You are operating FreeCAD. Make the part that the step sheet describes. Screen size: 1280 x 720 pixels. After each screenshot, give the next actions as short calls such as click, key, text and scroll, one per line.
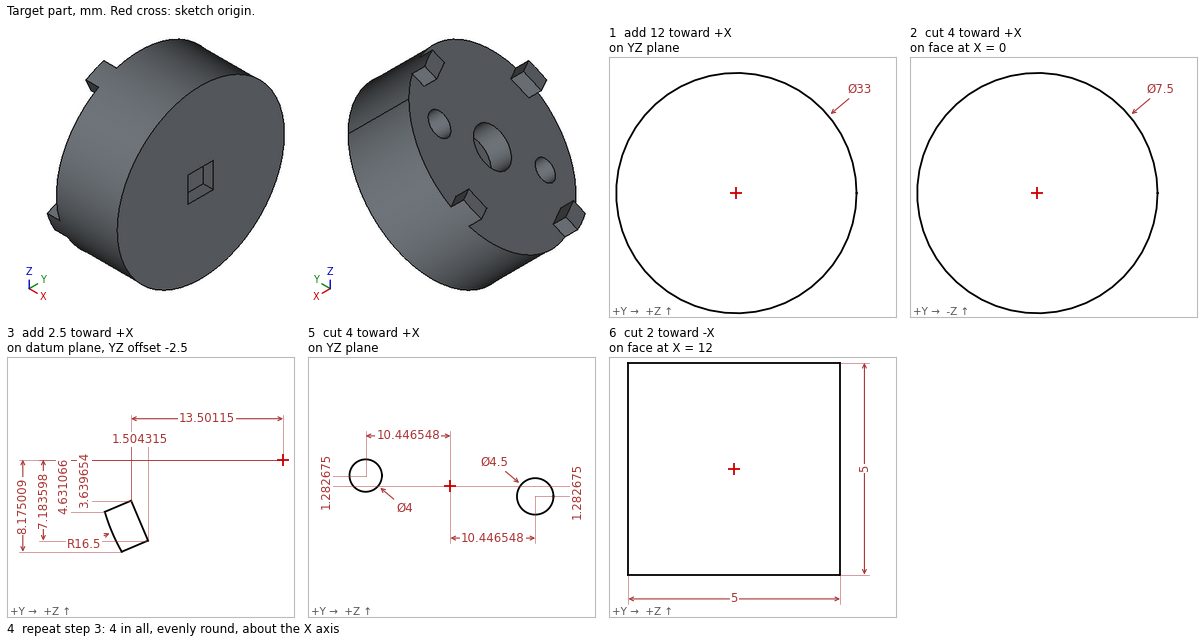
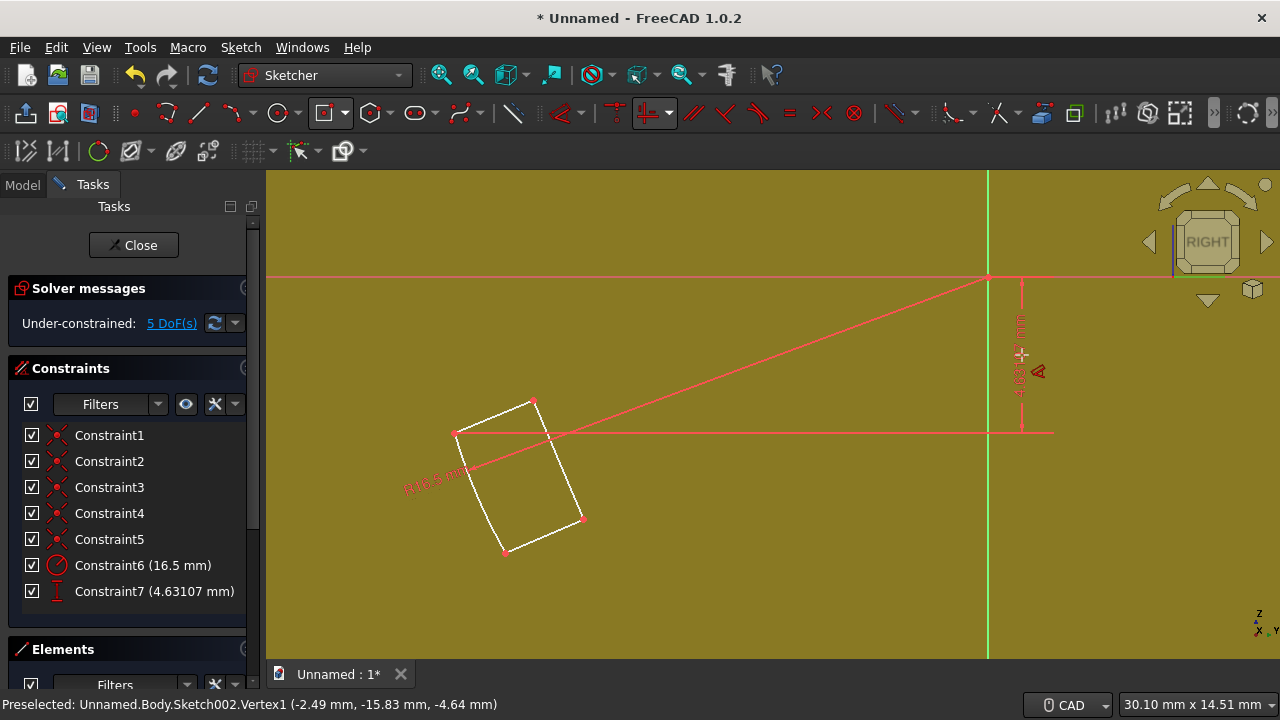
click(533, 400)
click(761, 243)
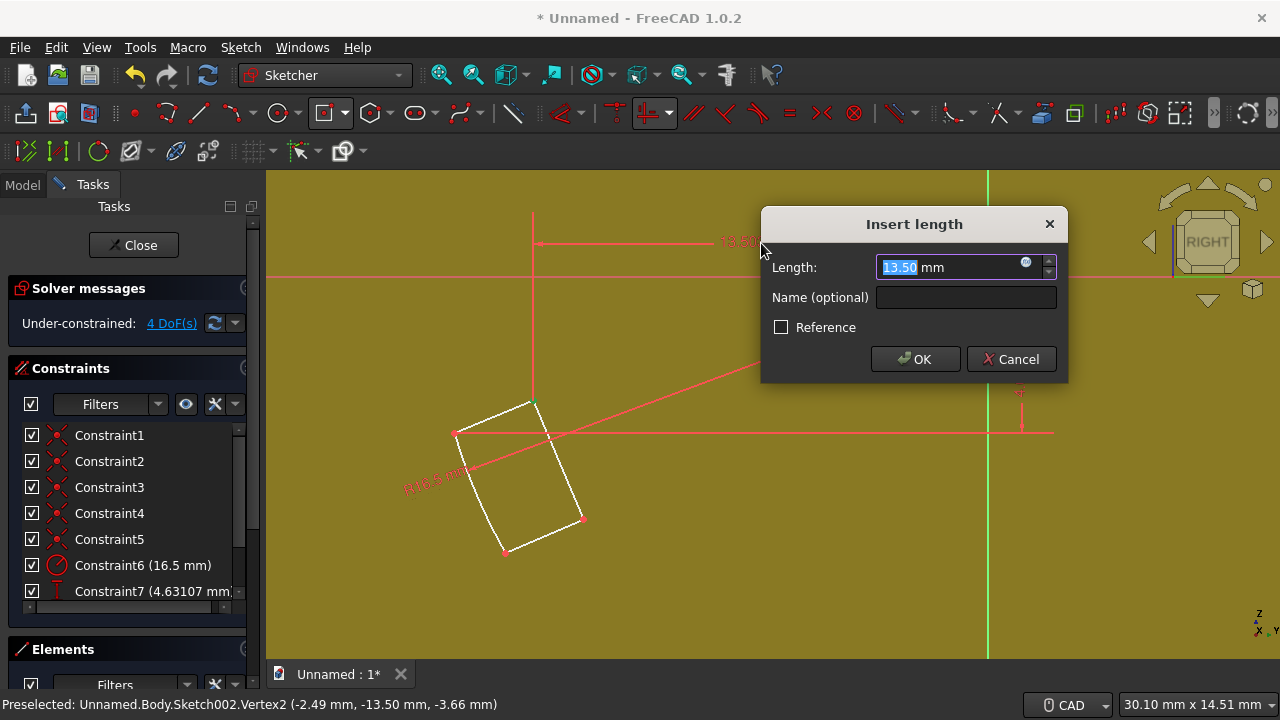
text(13.50115)
key(Return)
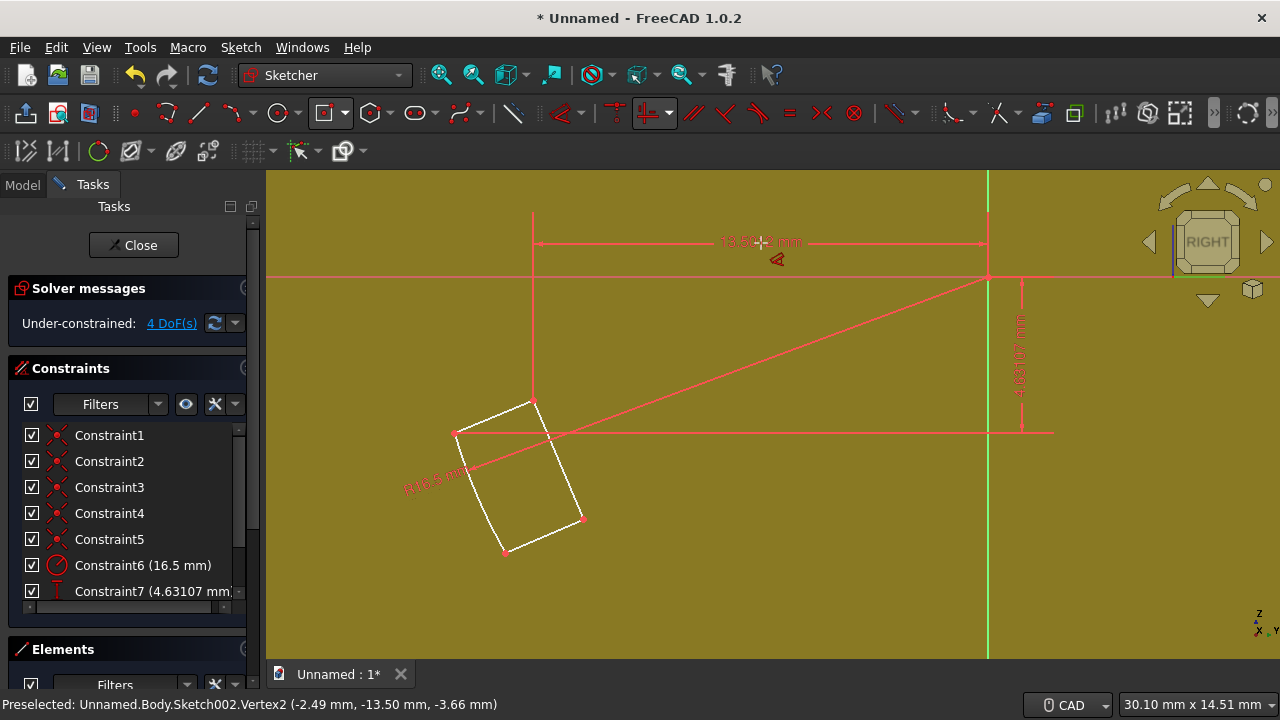
click(533, 400)
click(1022, 310)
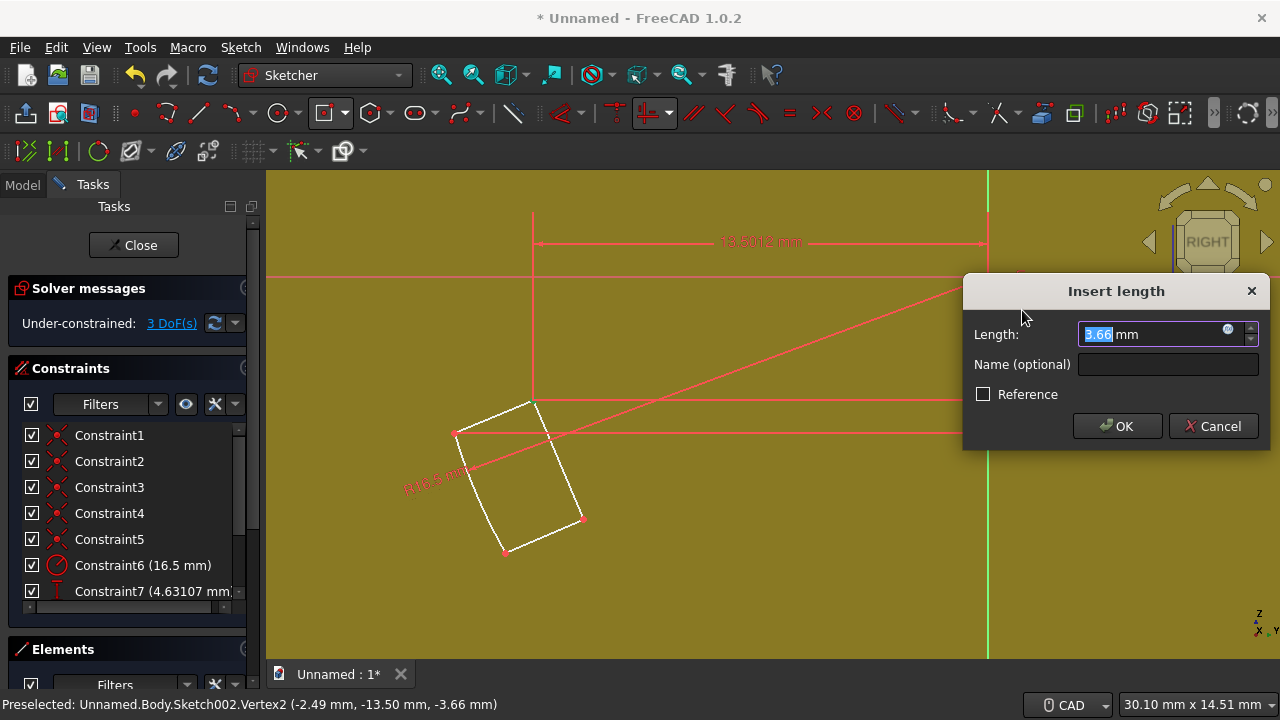
text(3.639654)
key(Return)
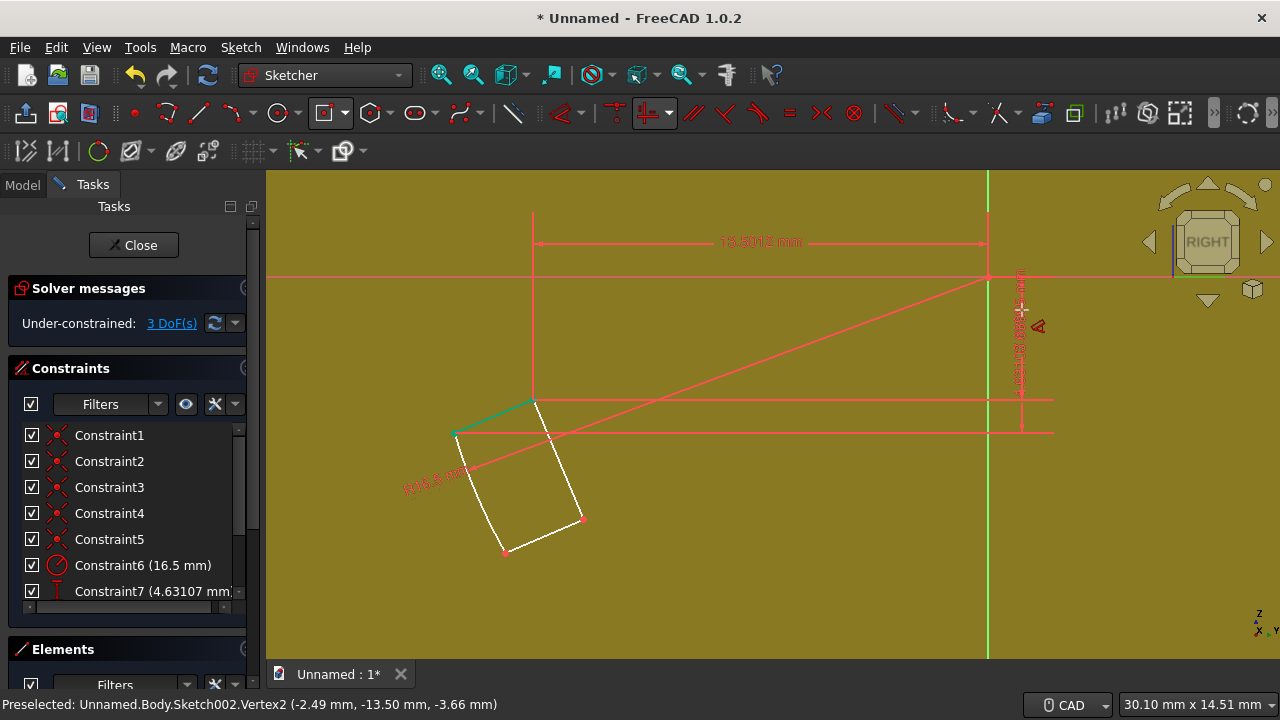
click(584, 520)
click(1022, 398)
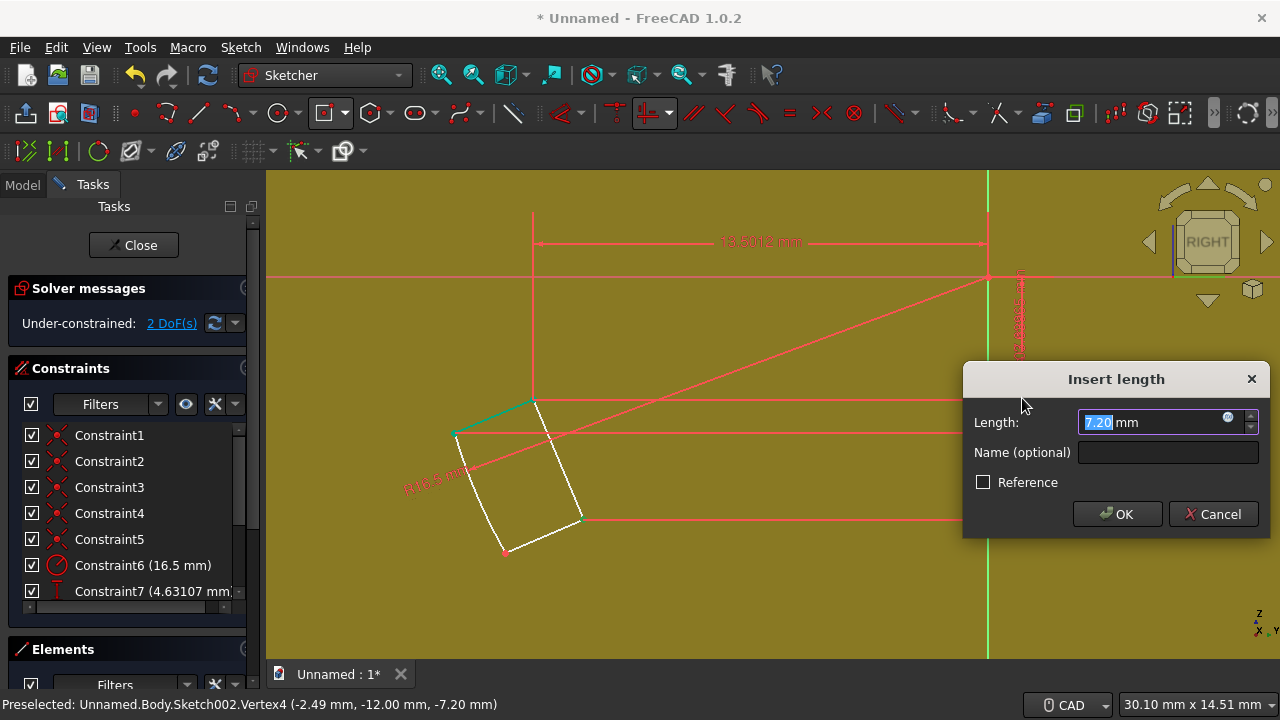
text(7.183598)
key(Return)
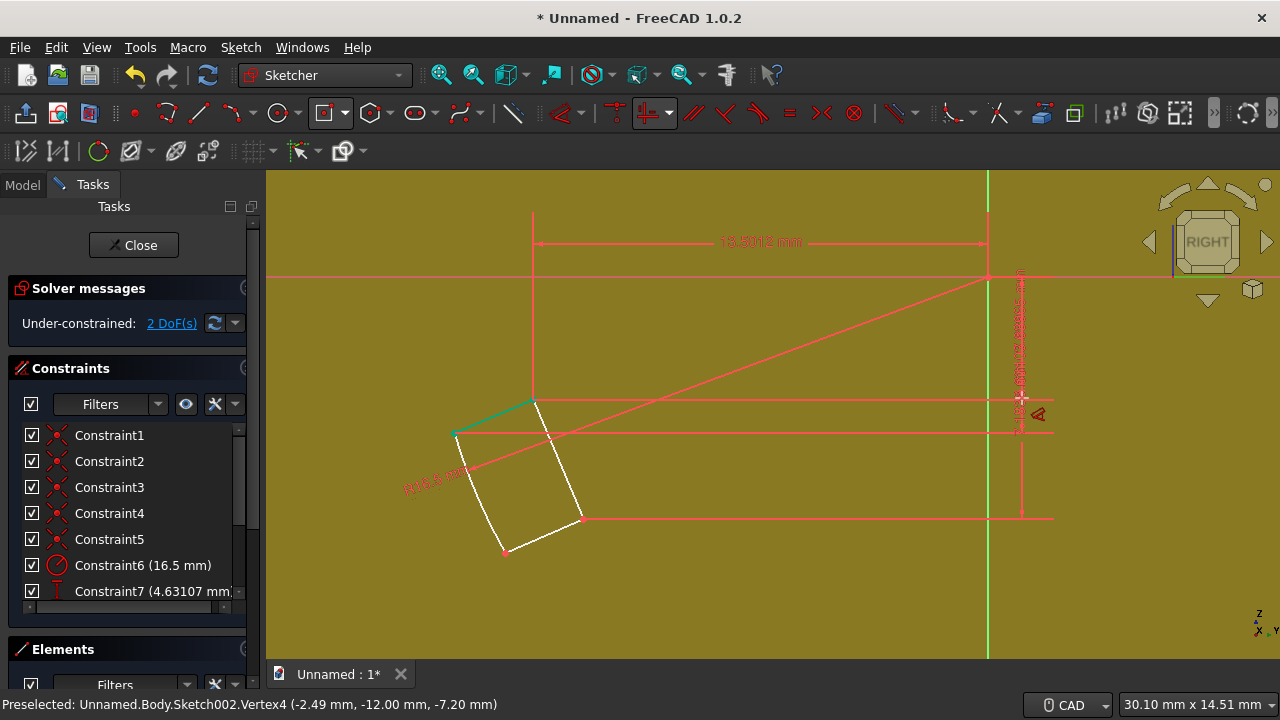
click(506, 553)
click(1022, 479)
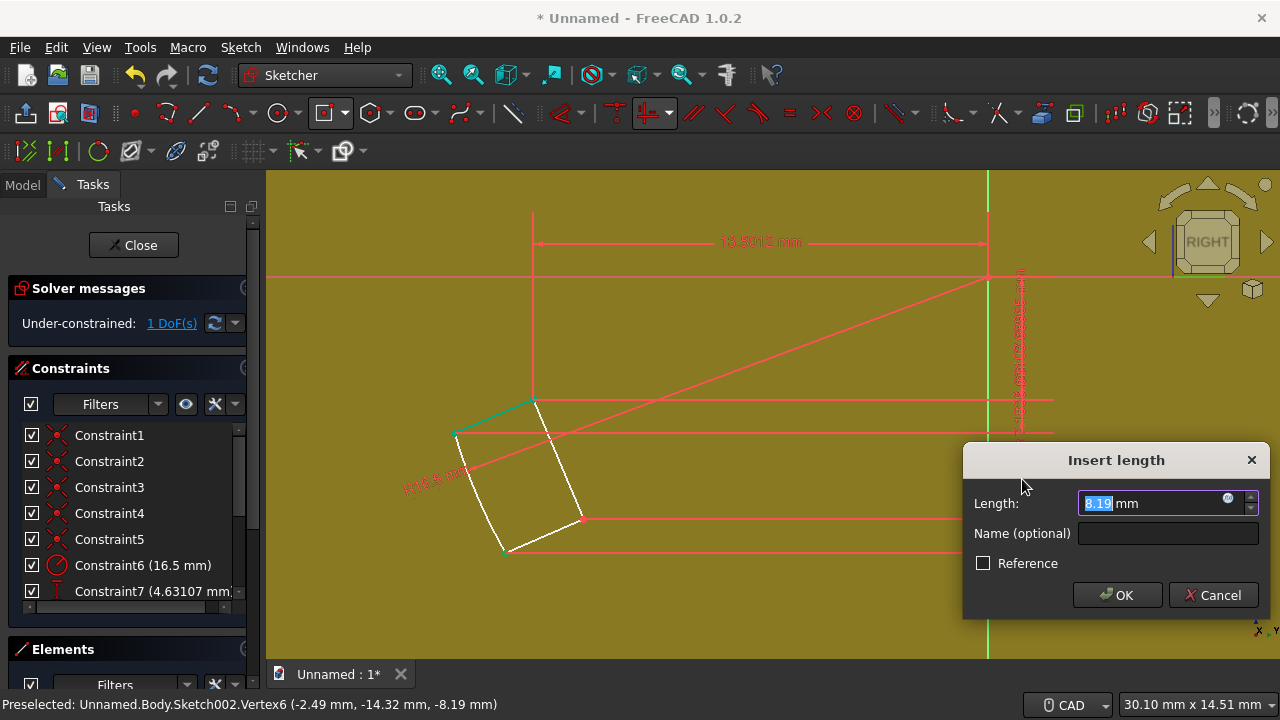
text(8.175009)
key(Return)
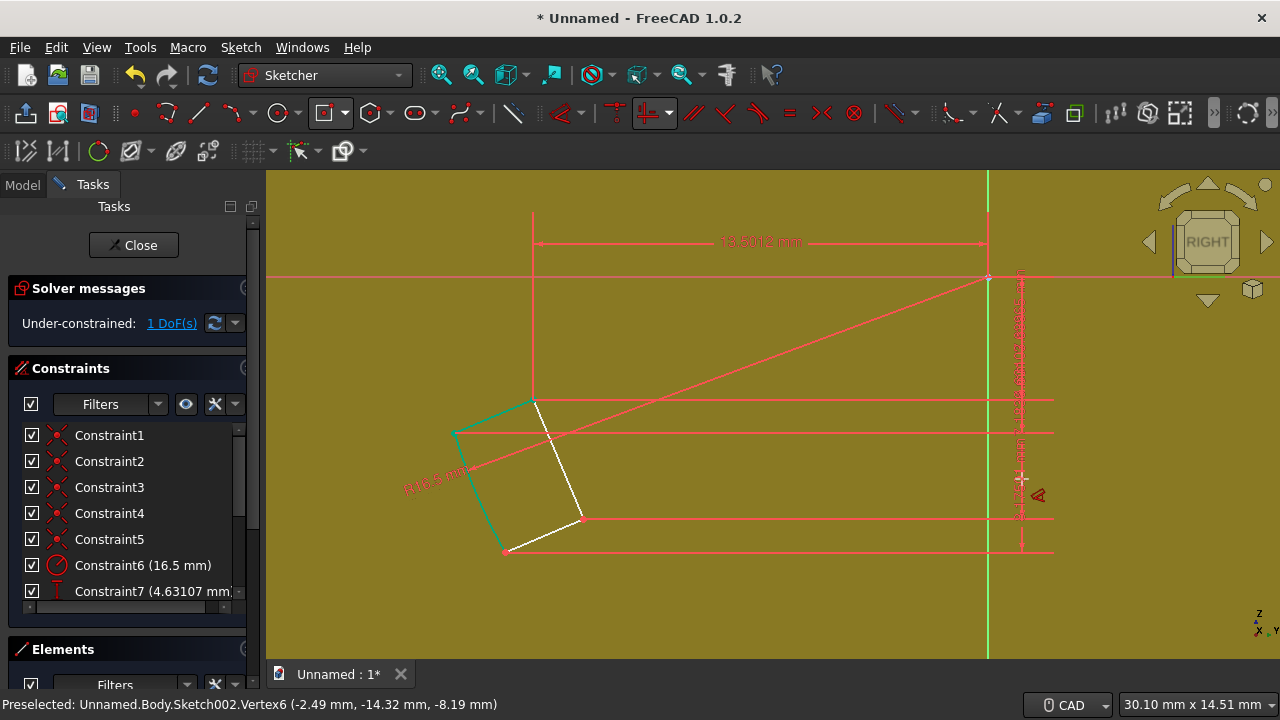
click(548, 436)
click(559, 366)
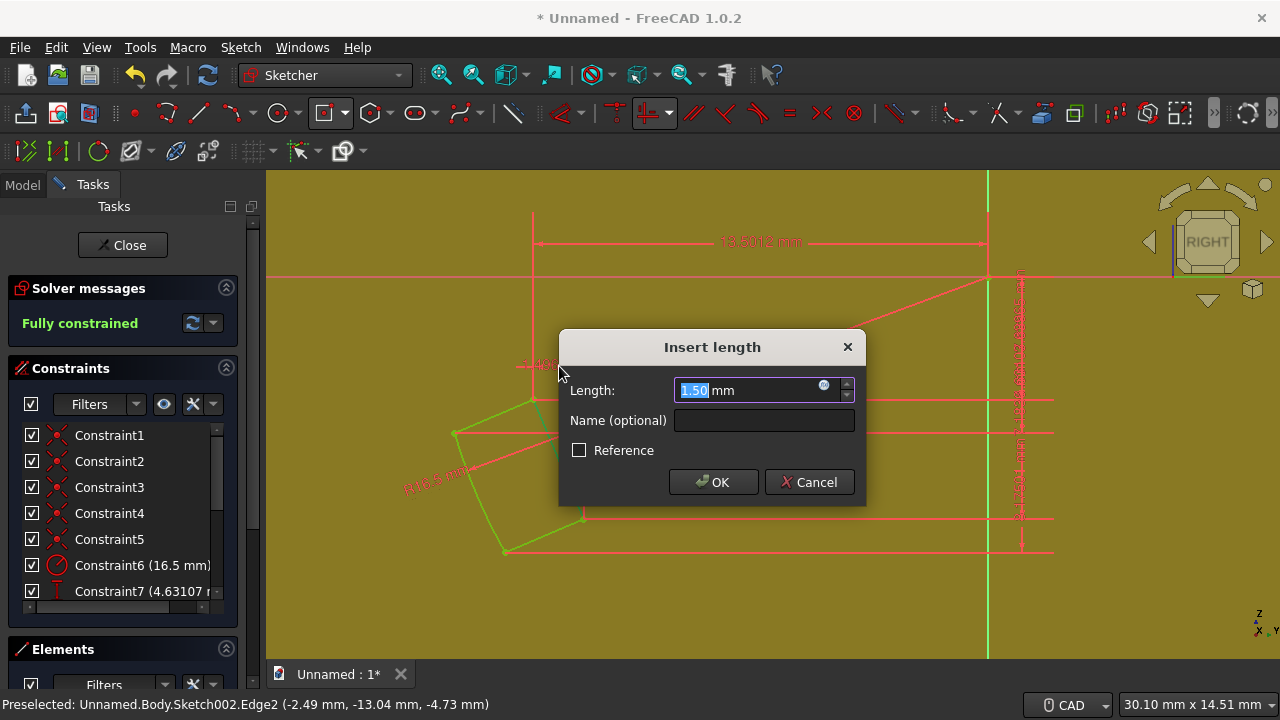
text(1.504315)
key(Return)
key(Escape)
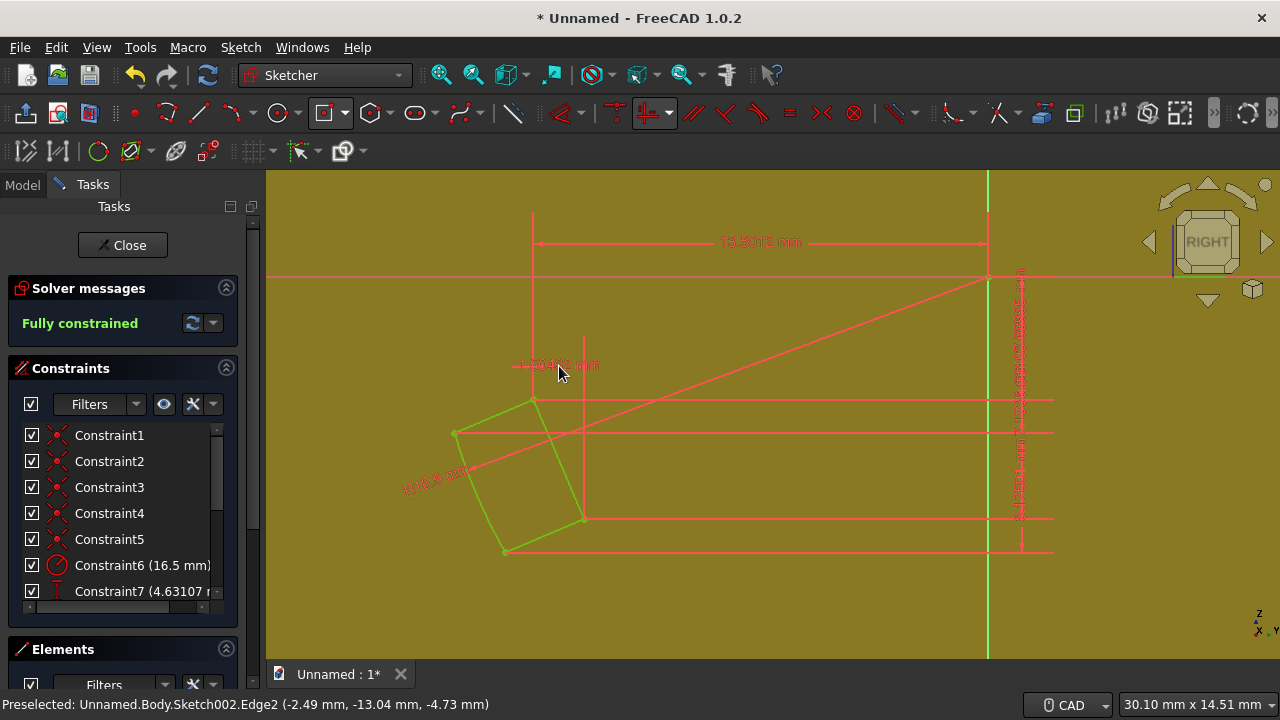
click(123, 245)